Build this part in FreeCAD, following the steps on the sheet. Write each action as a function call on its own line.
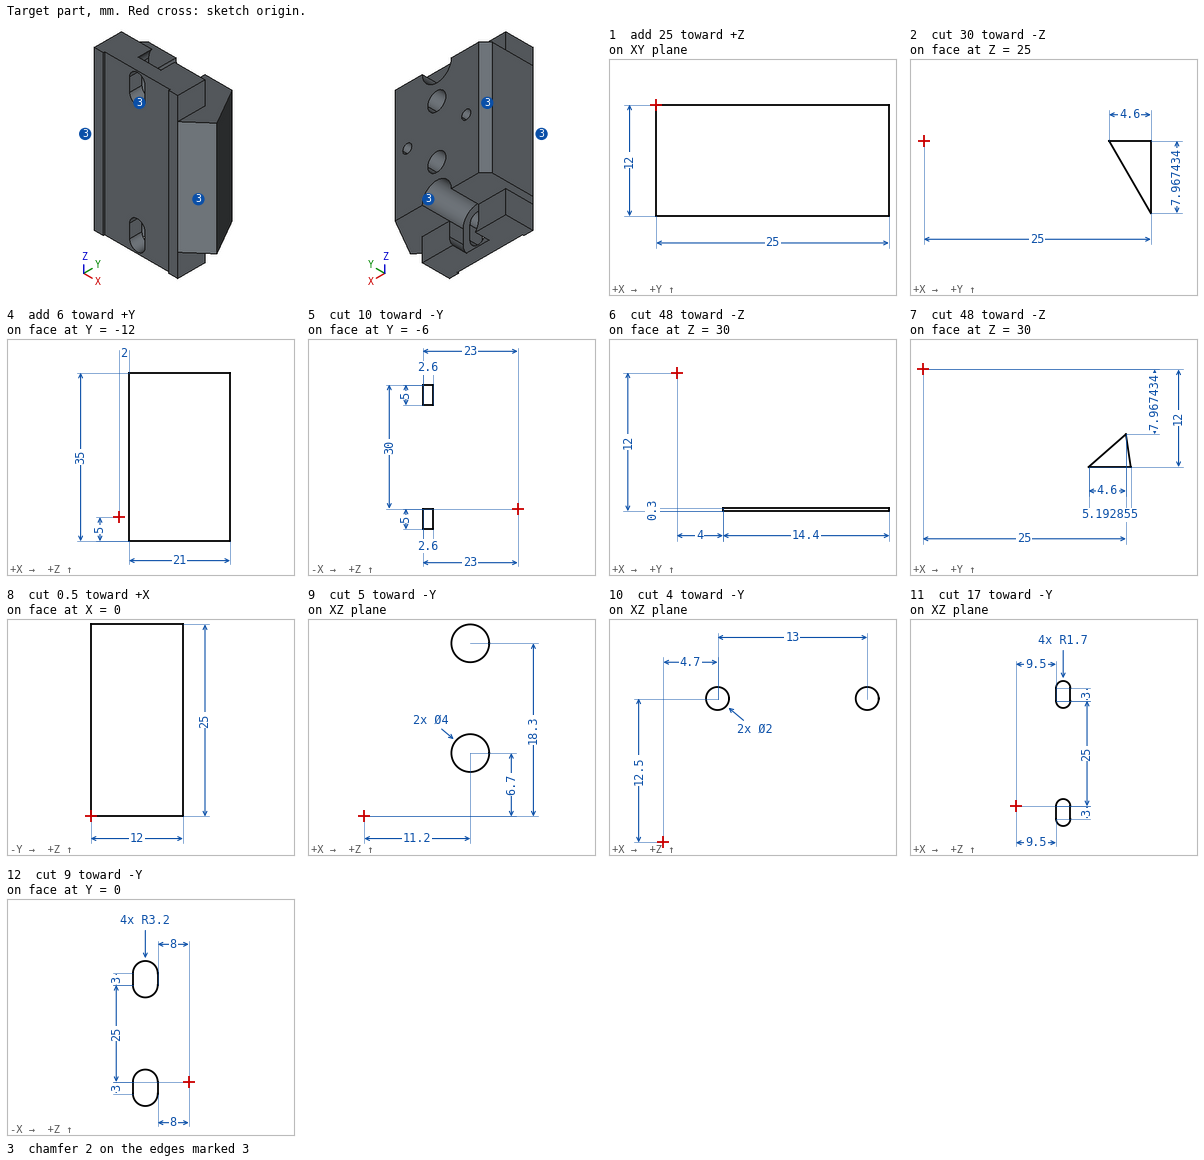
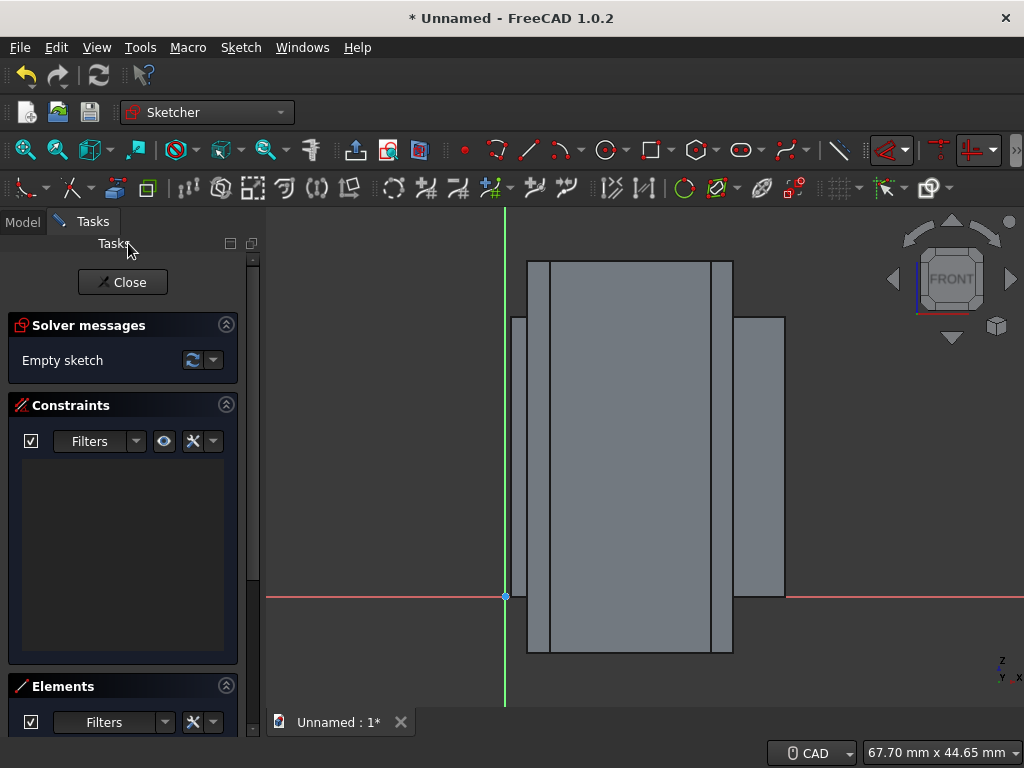
click(420, 150)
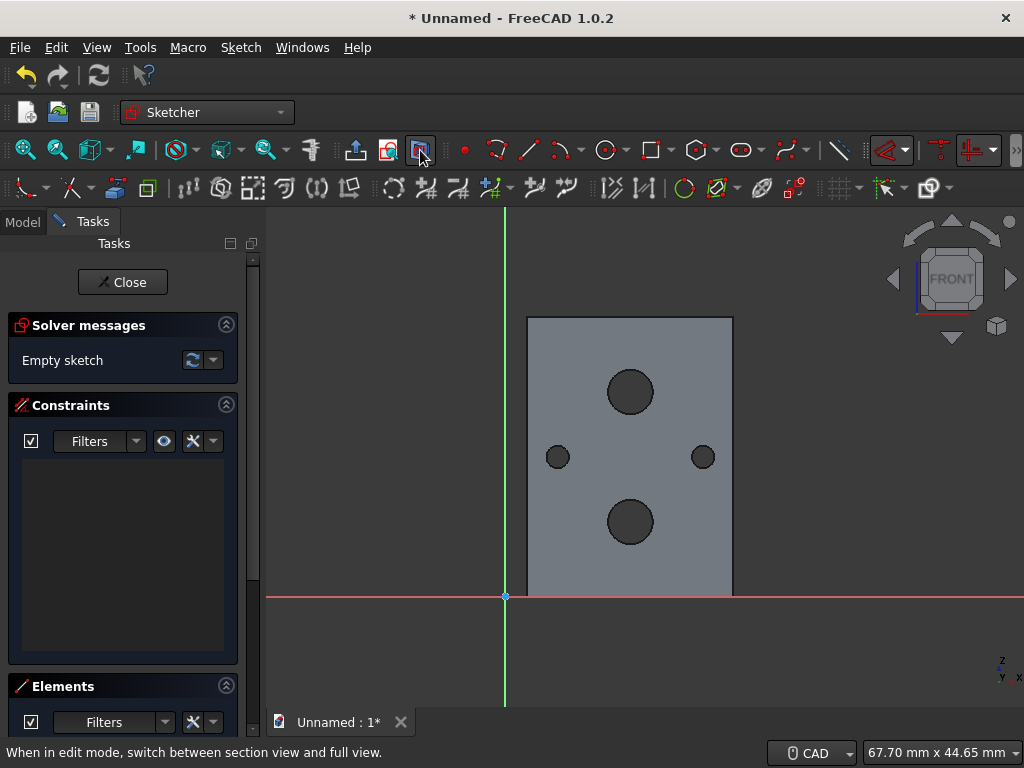
click(742, 150)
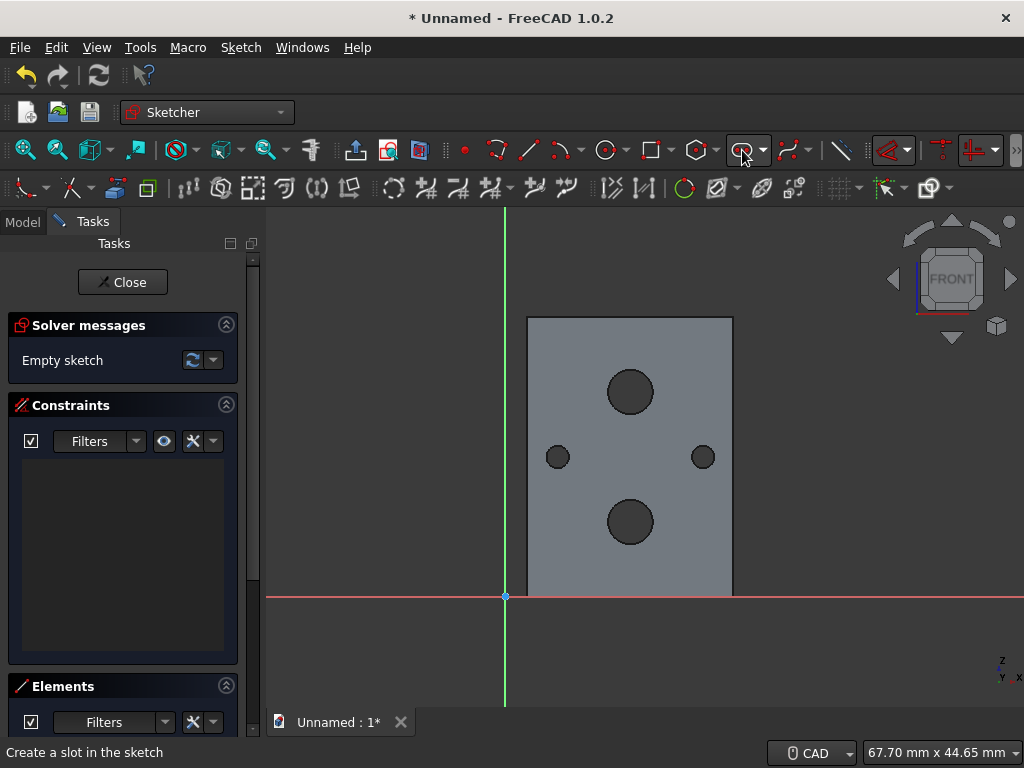
click(630, 317)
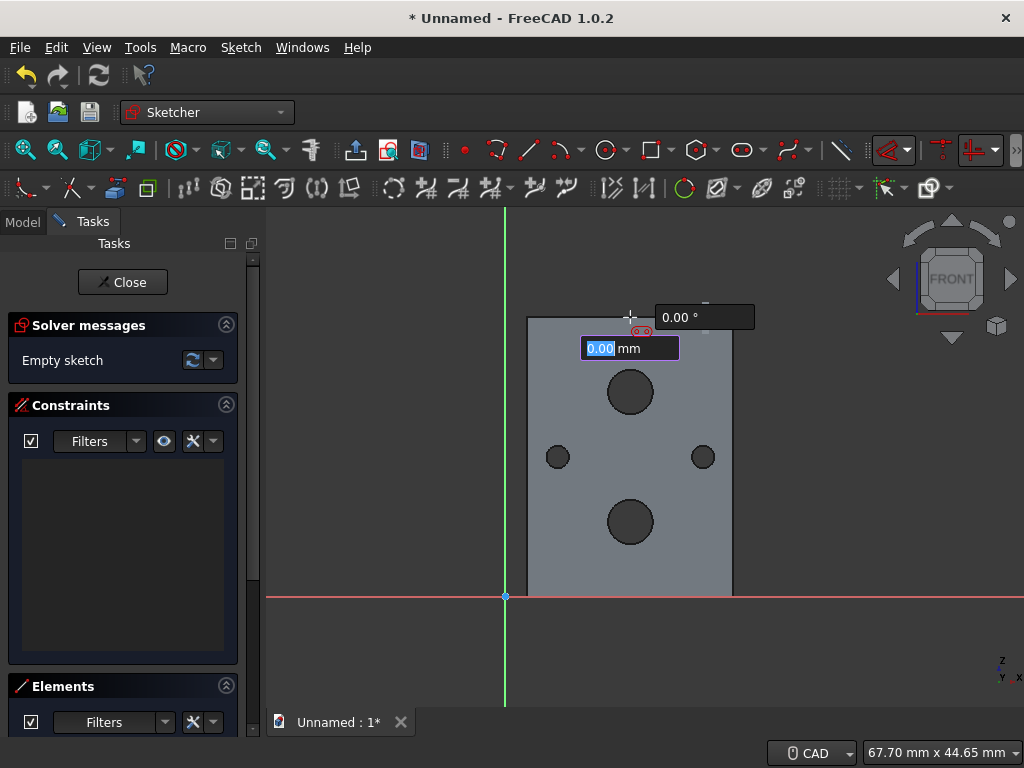
click(630, 283)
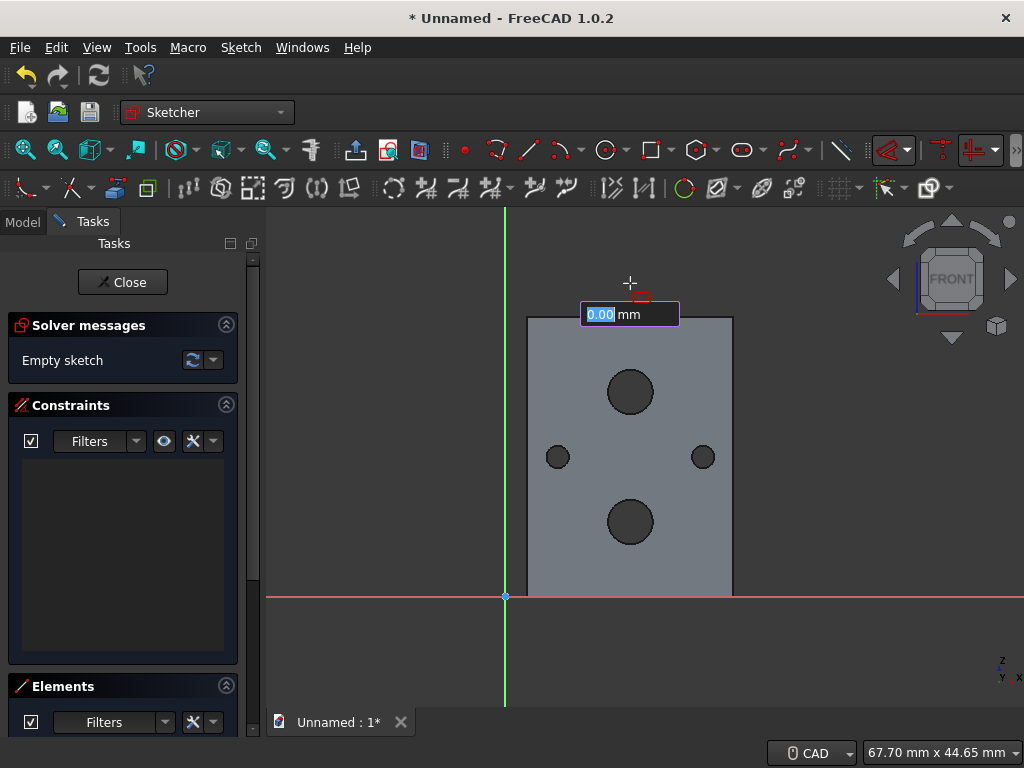
click(649, 300)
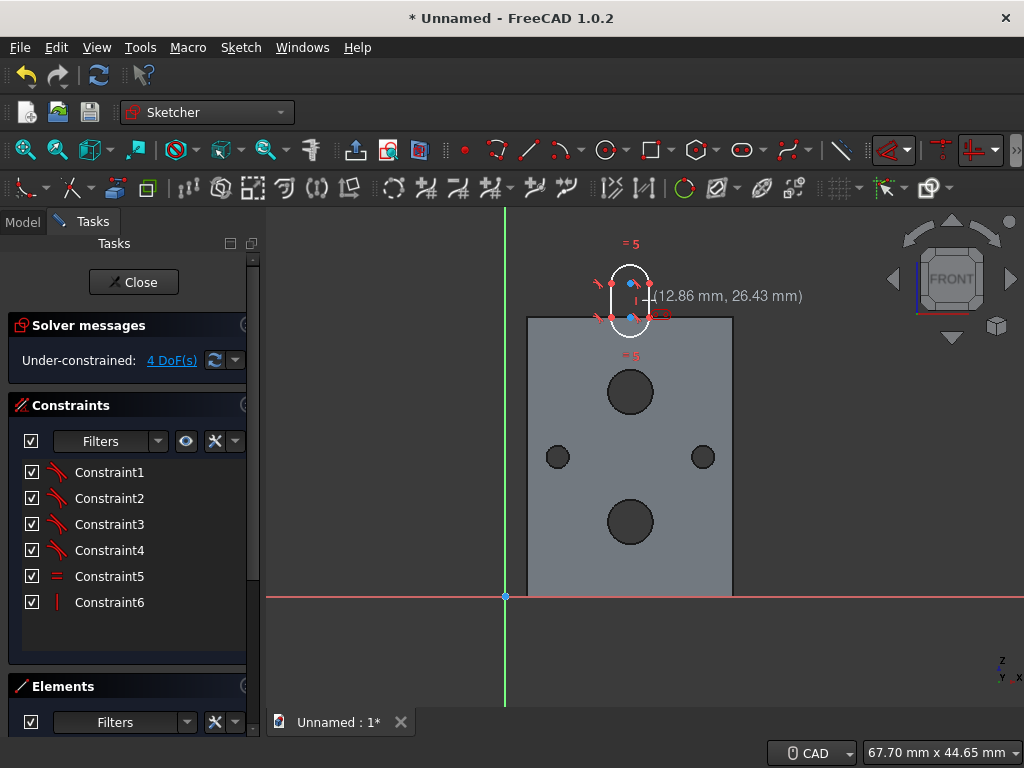
click(630, 631)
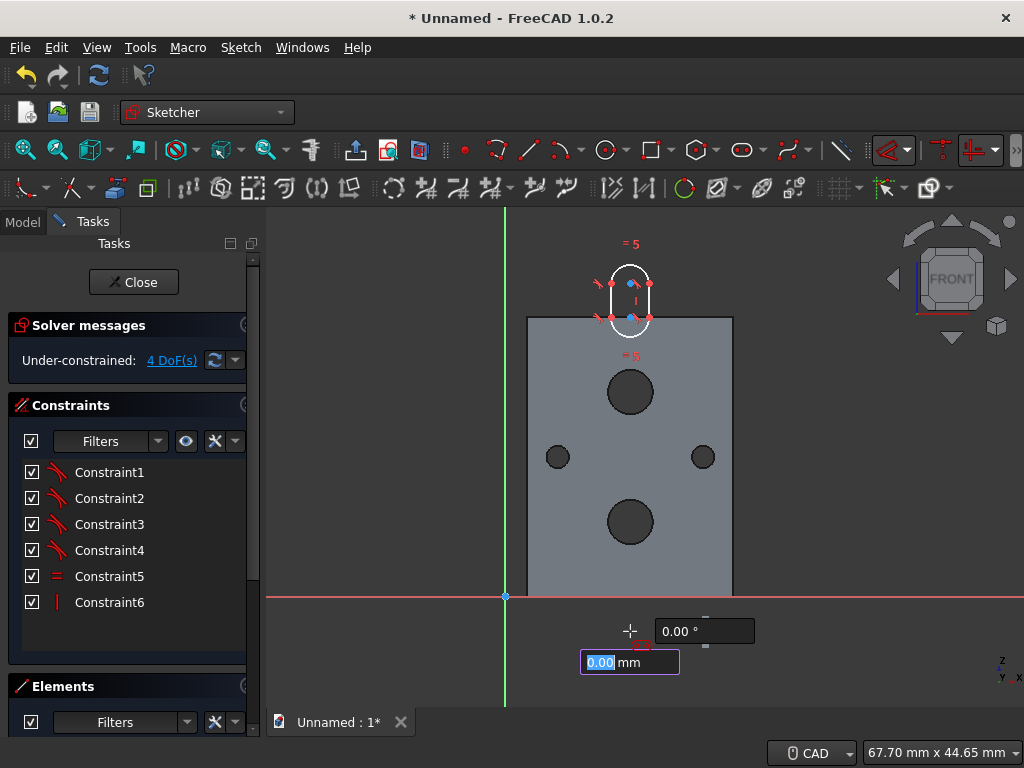
click(630, 597)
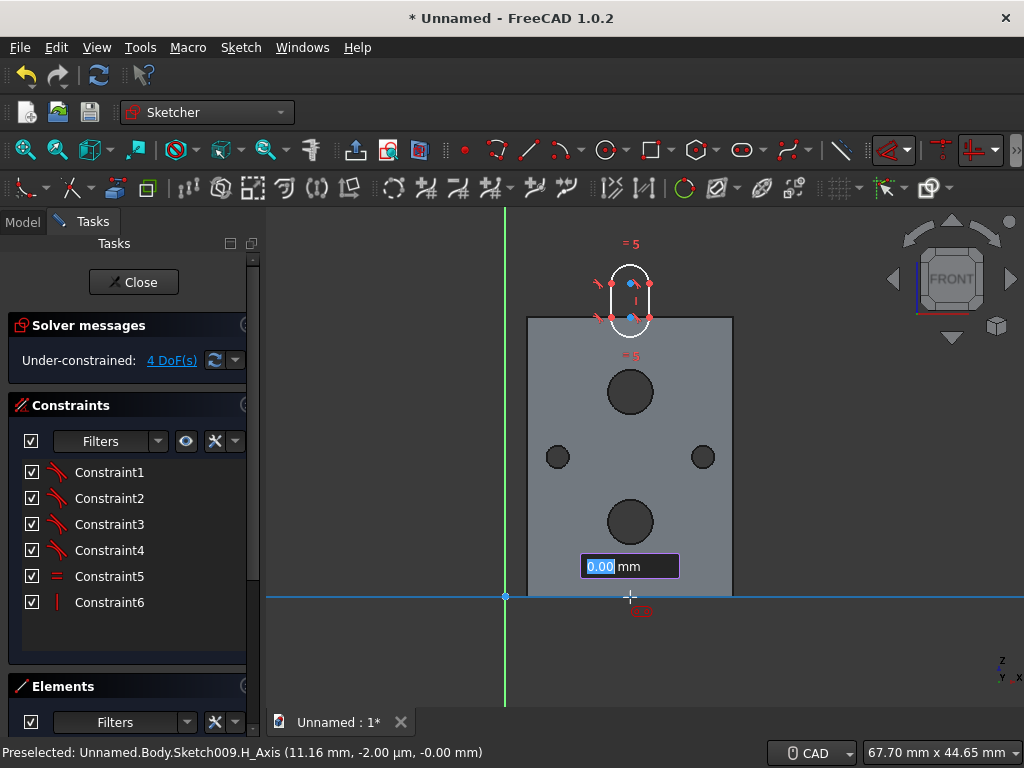
click(649, 614)
key(Escape)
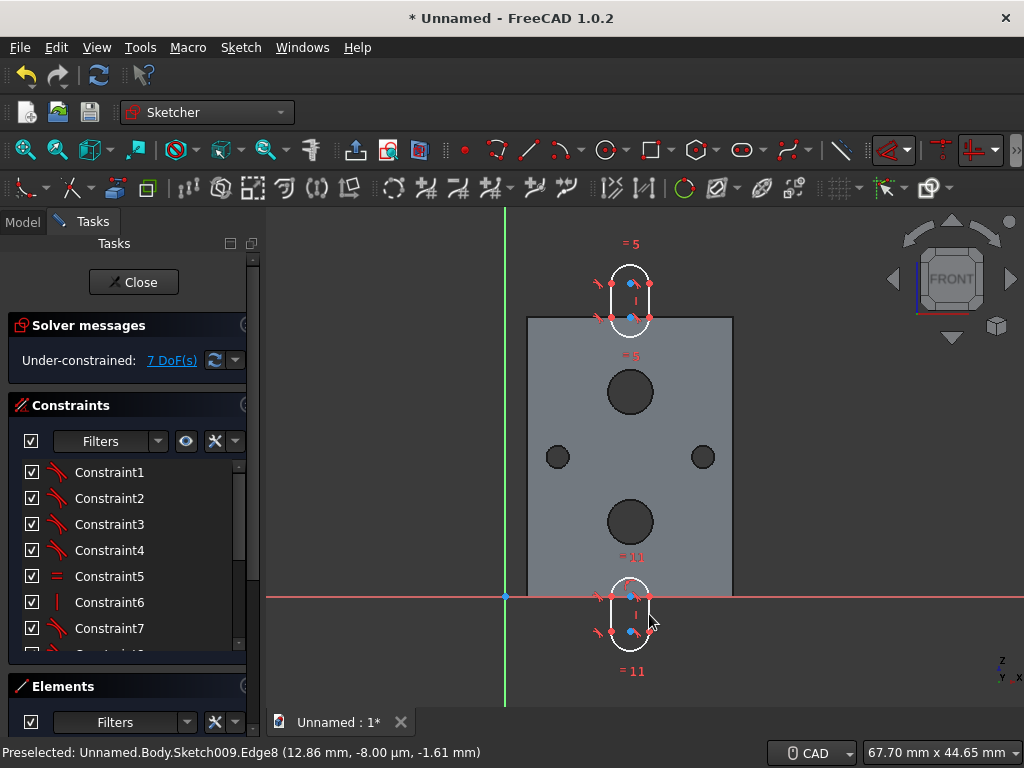
click(619, 333)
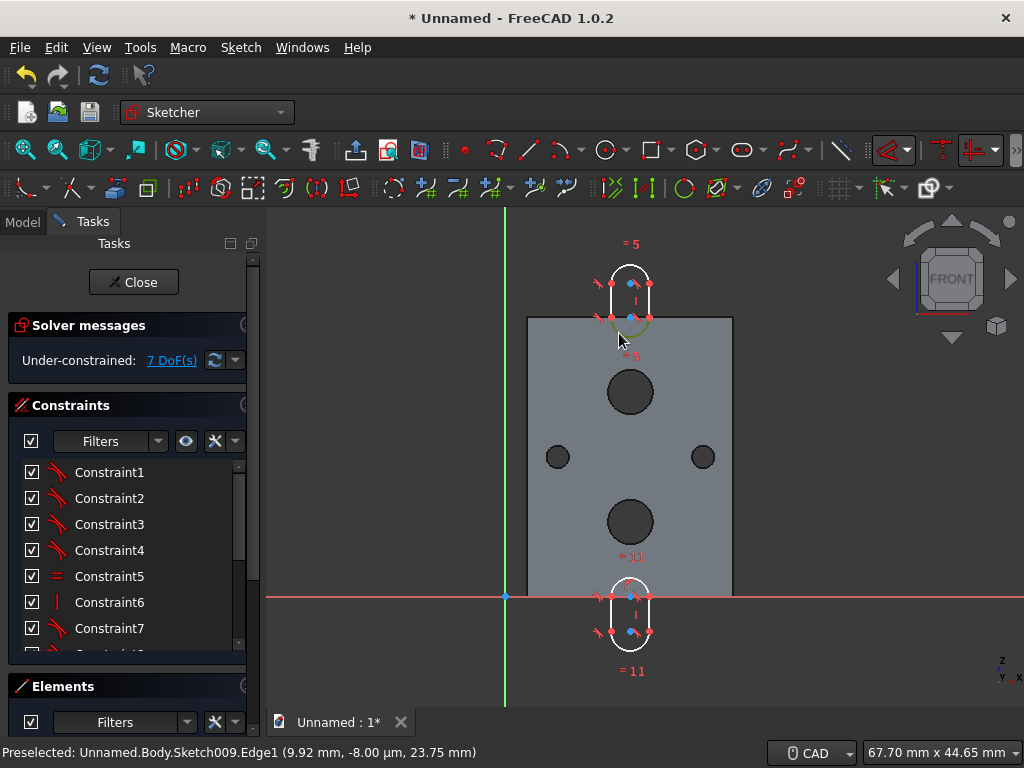
click(619, 647)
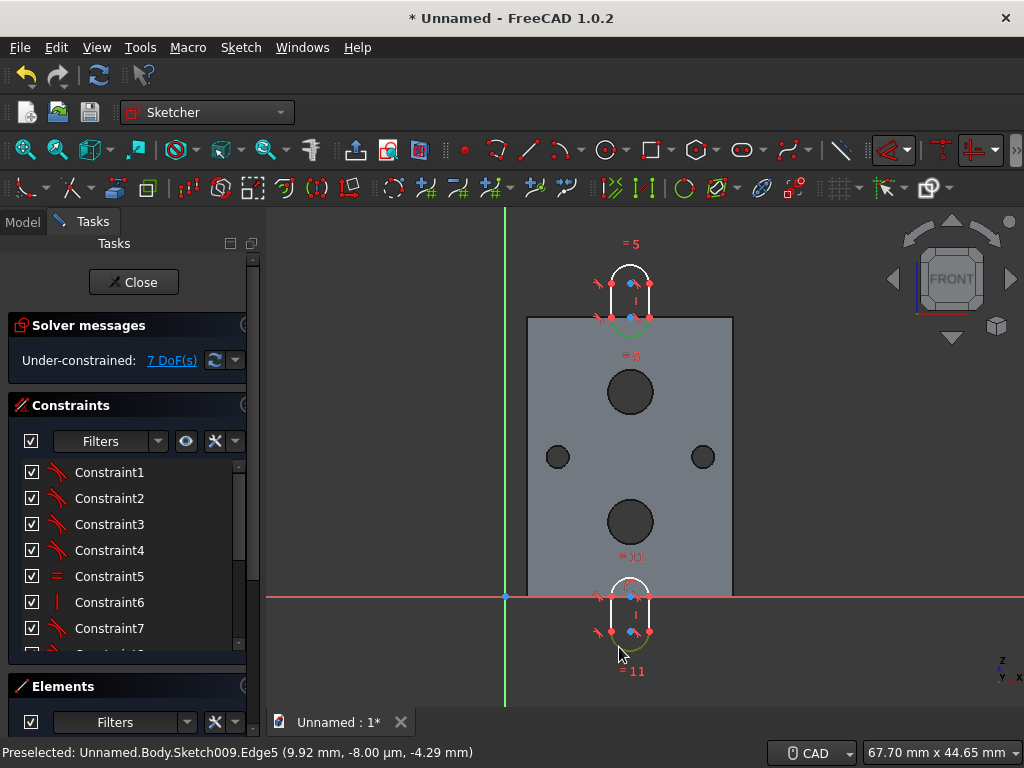
key(e)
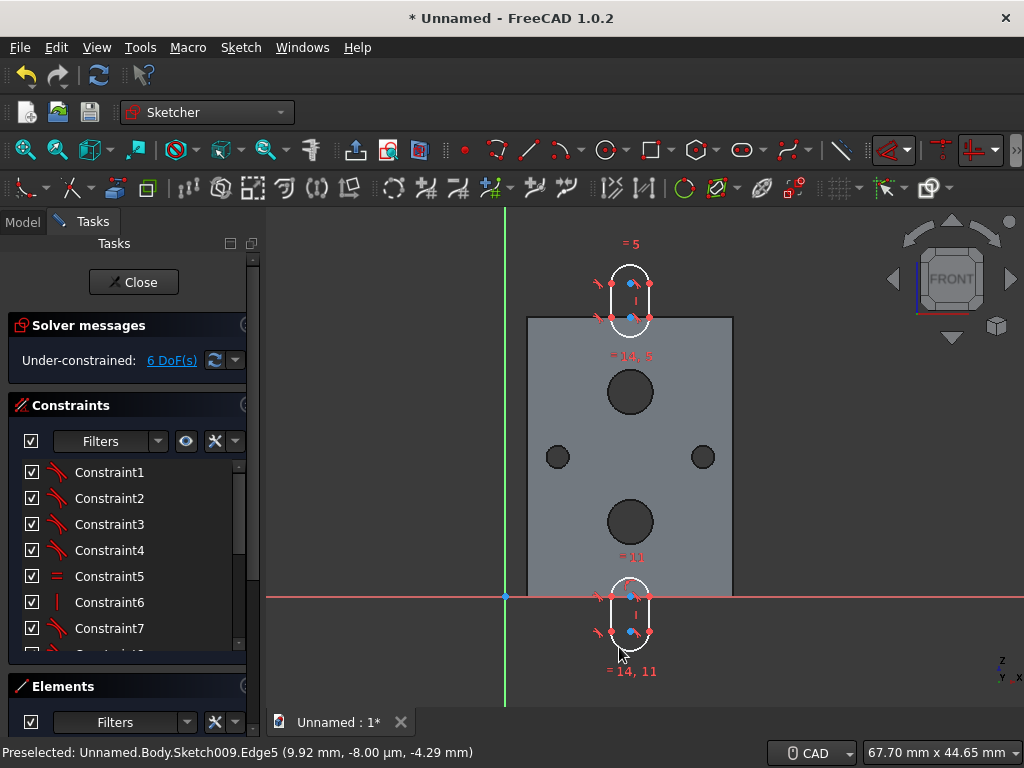
scroll(619, 333, up, 4)